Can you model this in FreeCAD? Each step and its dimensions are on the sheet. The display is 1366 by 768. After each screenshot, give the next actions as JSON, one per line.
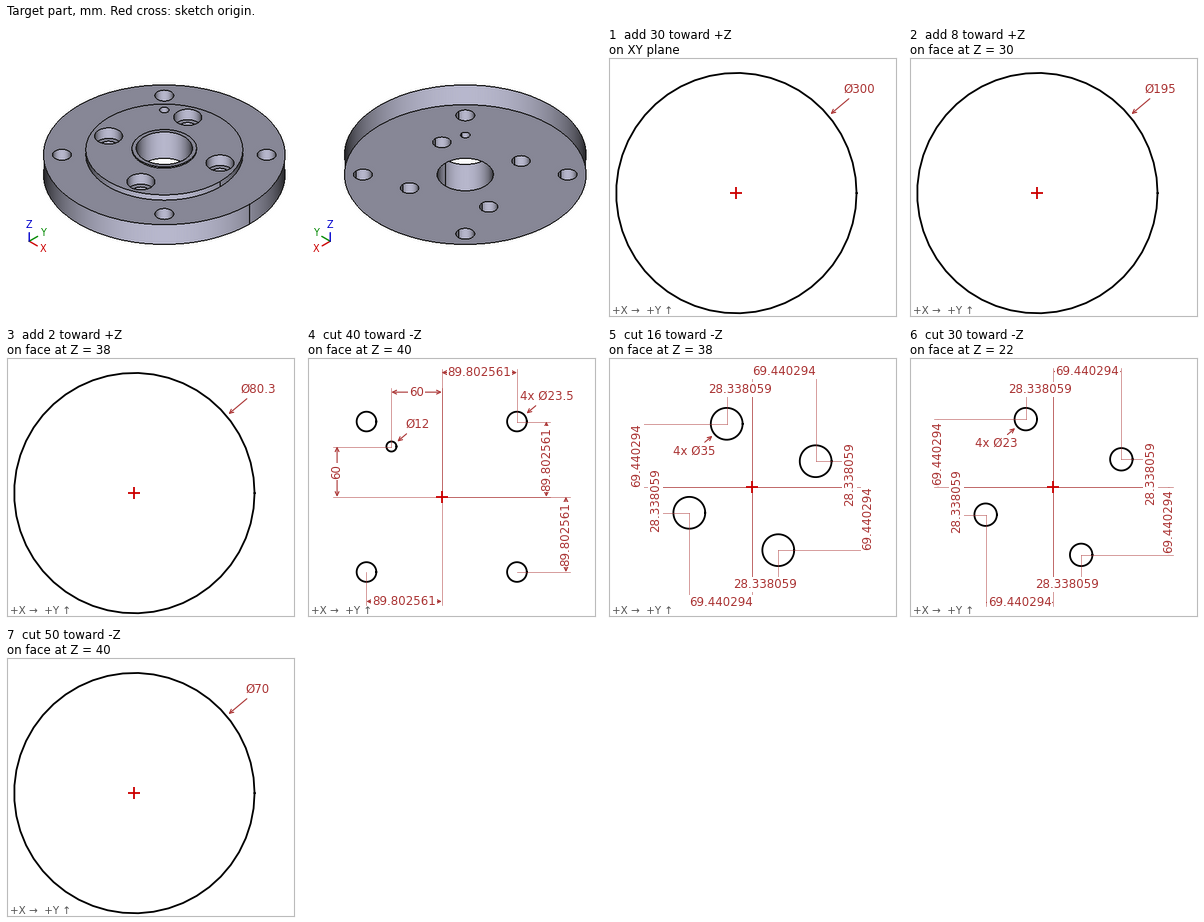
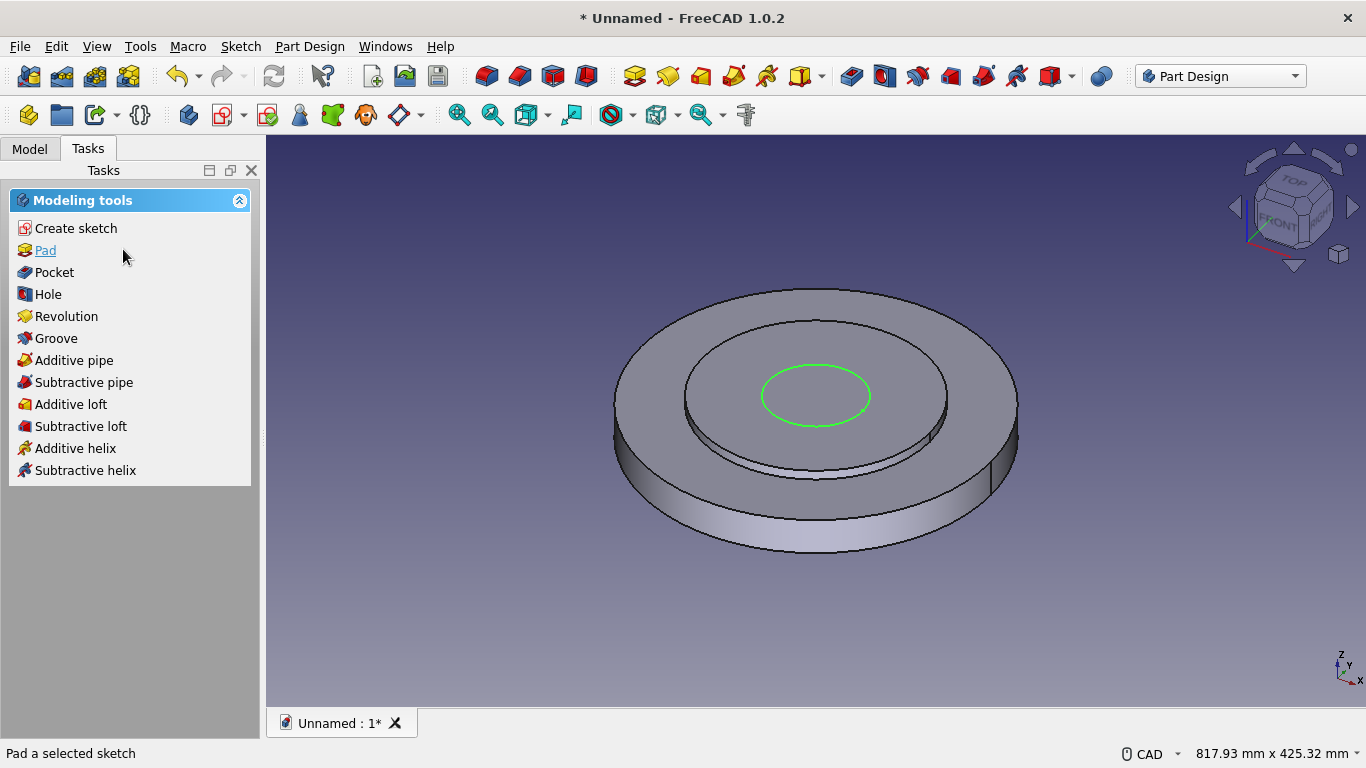
{"action": "left_click", "coordinate": [635, 76]}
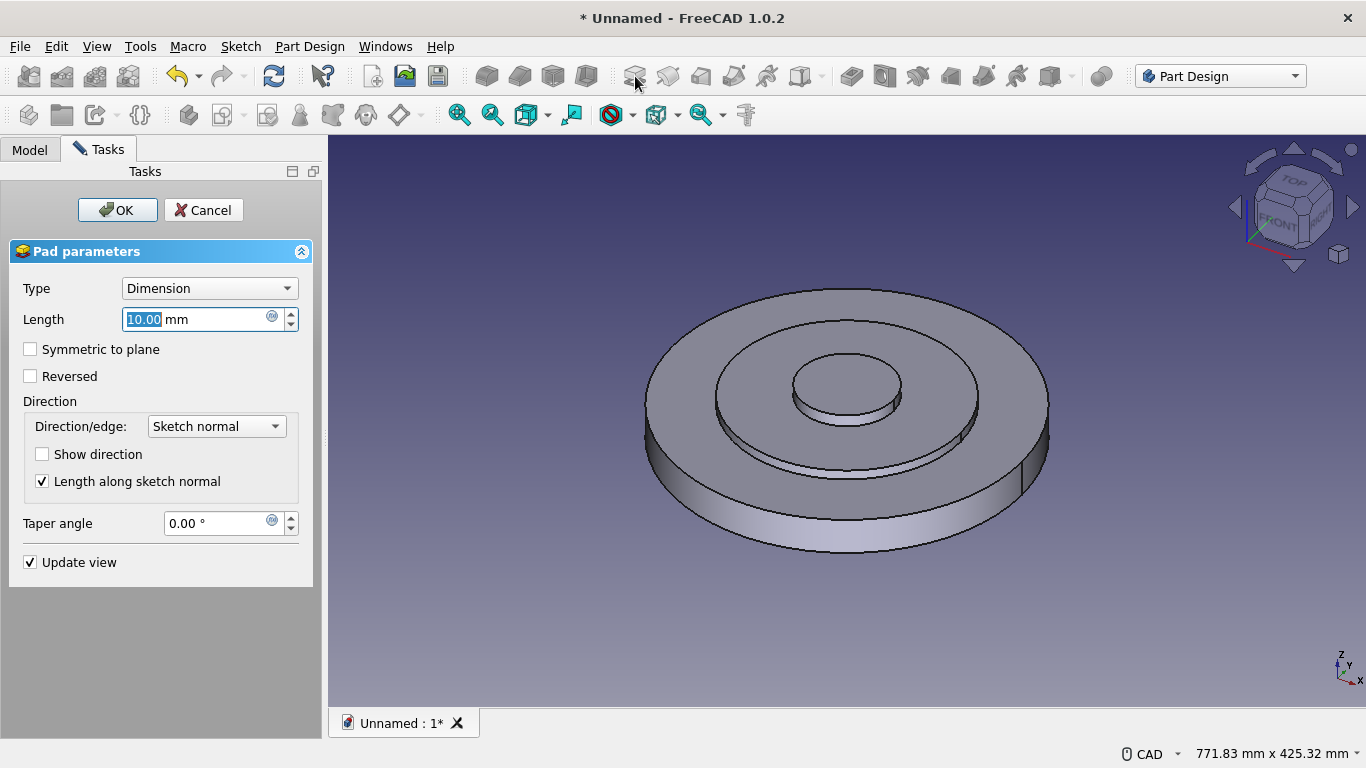
{"action": "type", "text": "2"}
{"action": "key", "text": "Tab"}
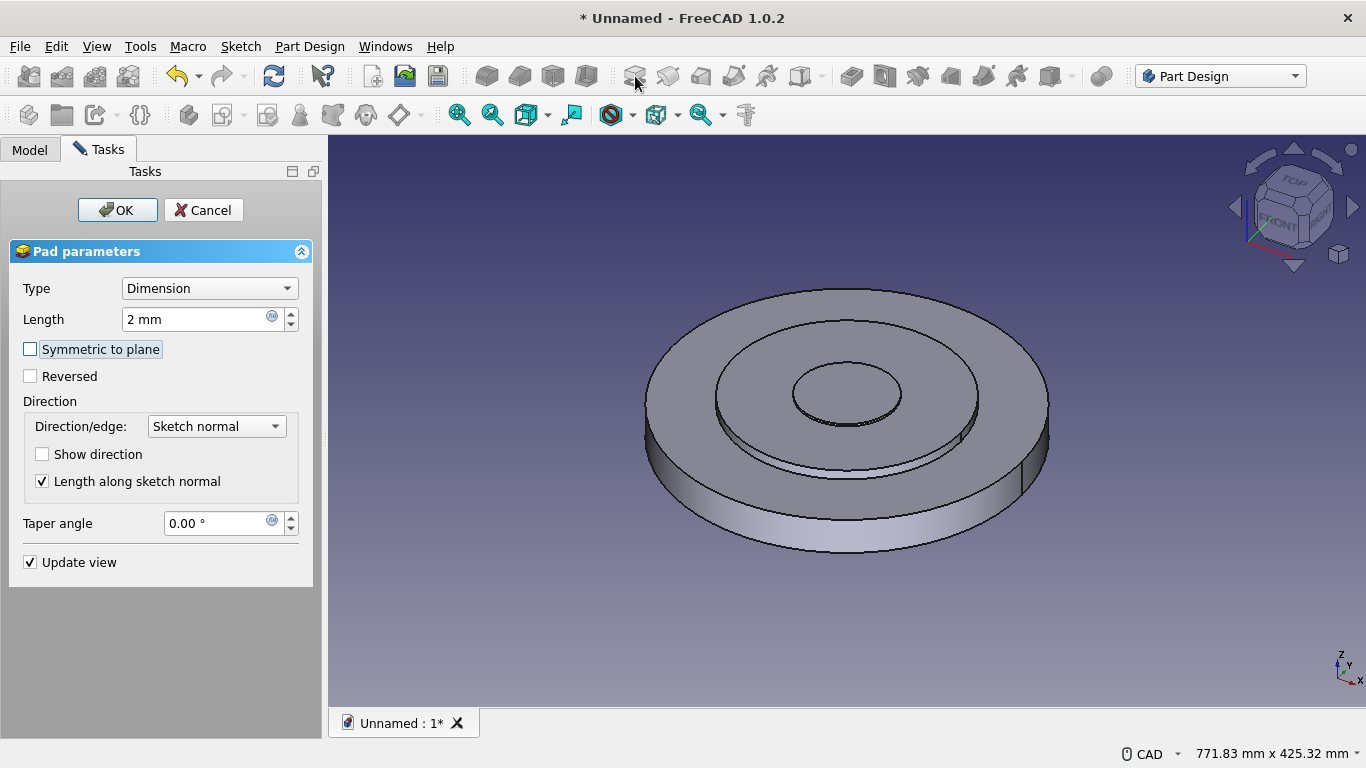
{"action": "left_click", "coordinate": [118, 210]}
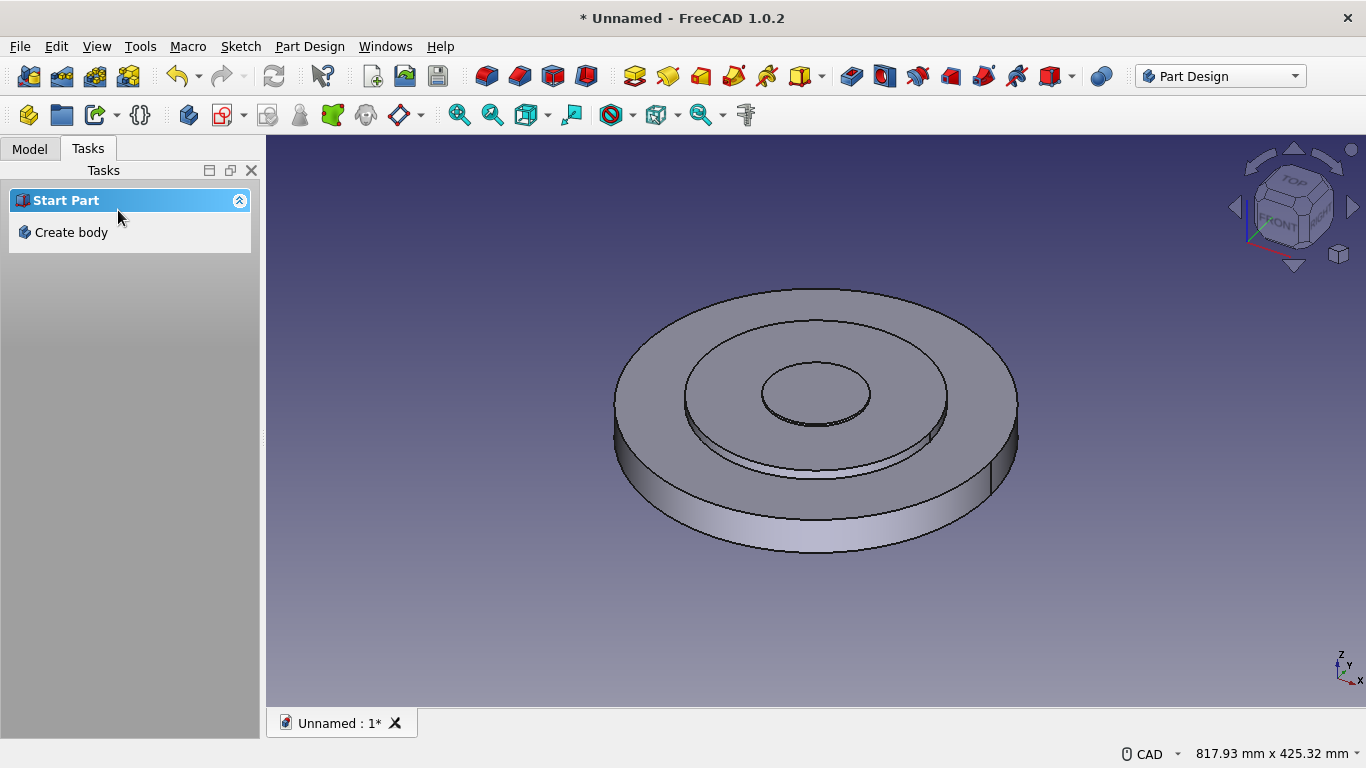
{"action": "left_click", "coordinate": [816, 392]}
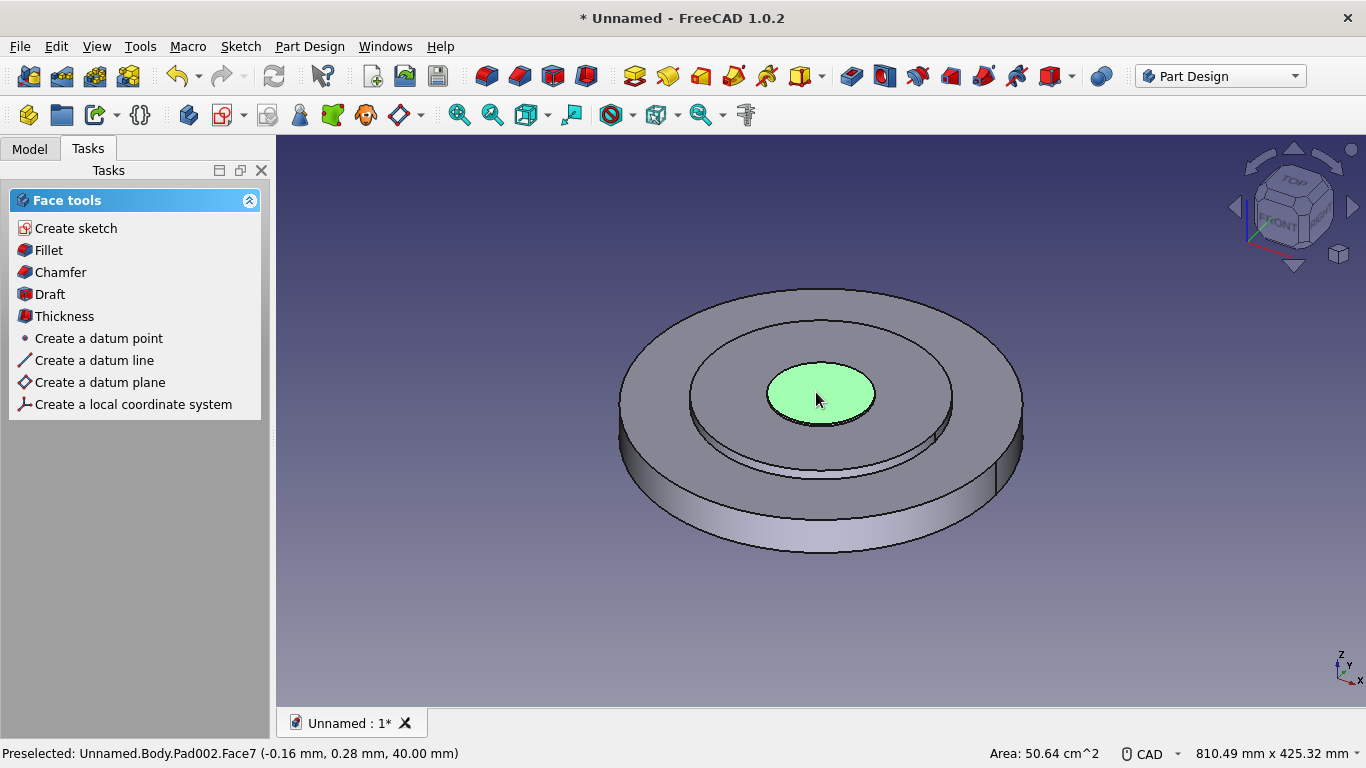
{"action": "left_click", "coordinate": [222, 116]}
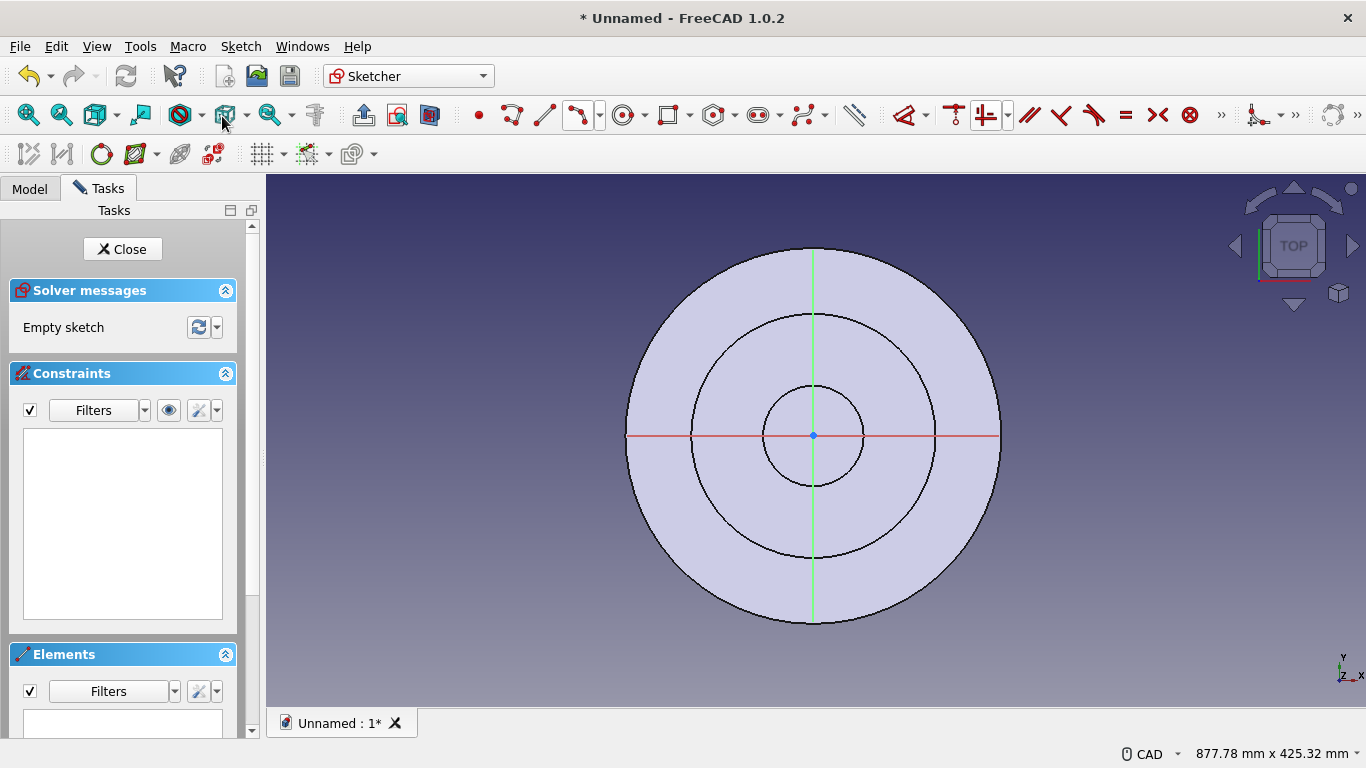
{"action": "left_click", "coordinate": [622, 116]}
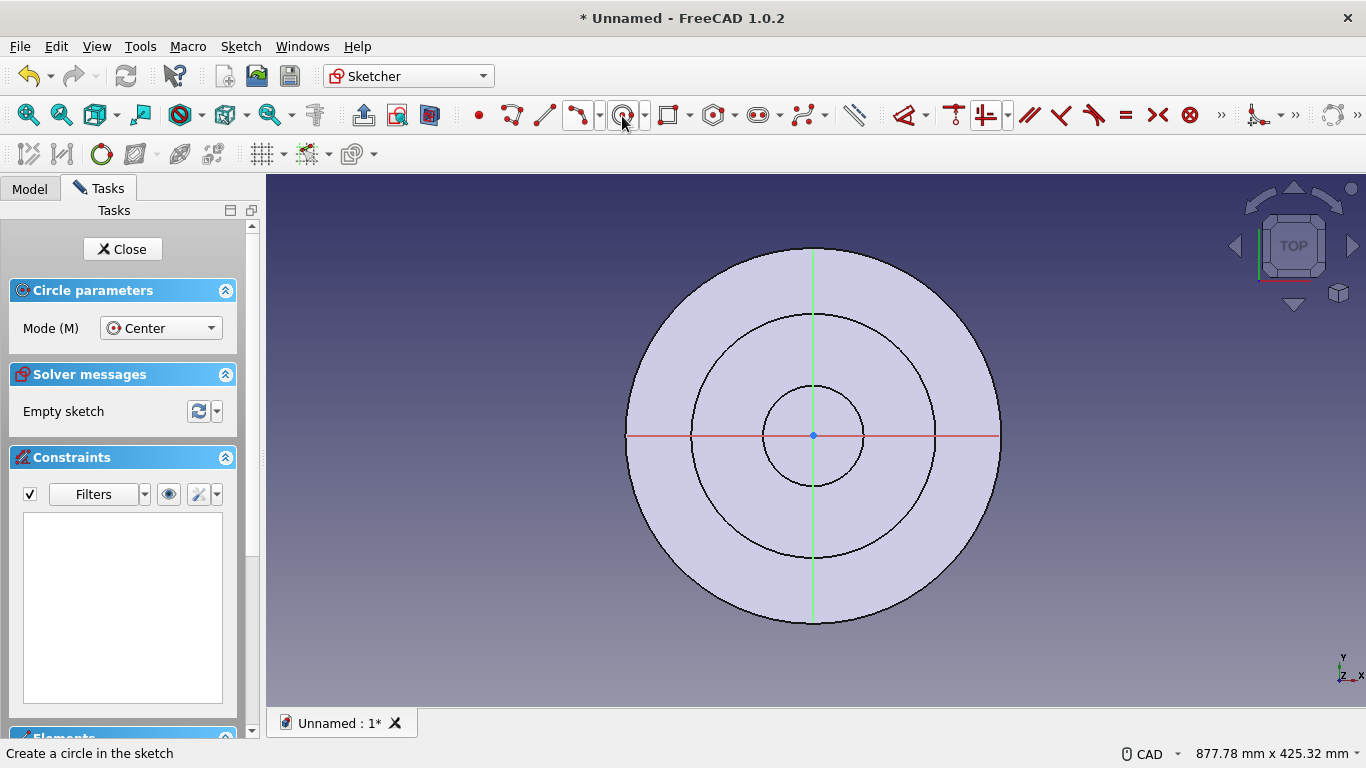
{"action": "scroll", "coordinate": [738, 361], "scroll_direction": "up", "scroll_amount": 6}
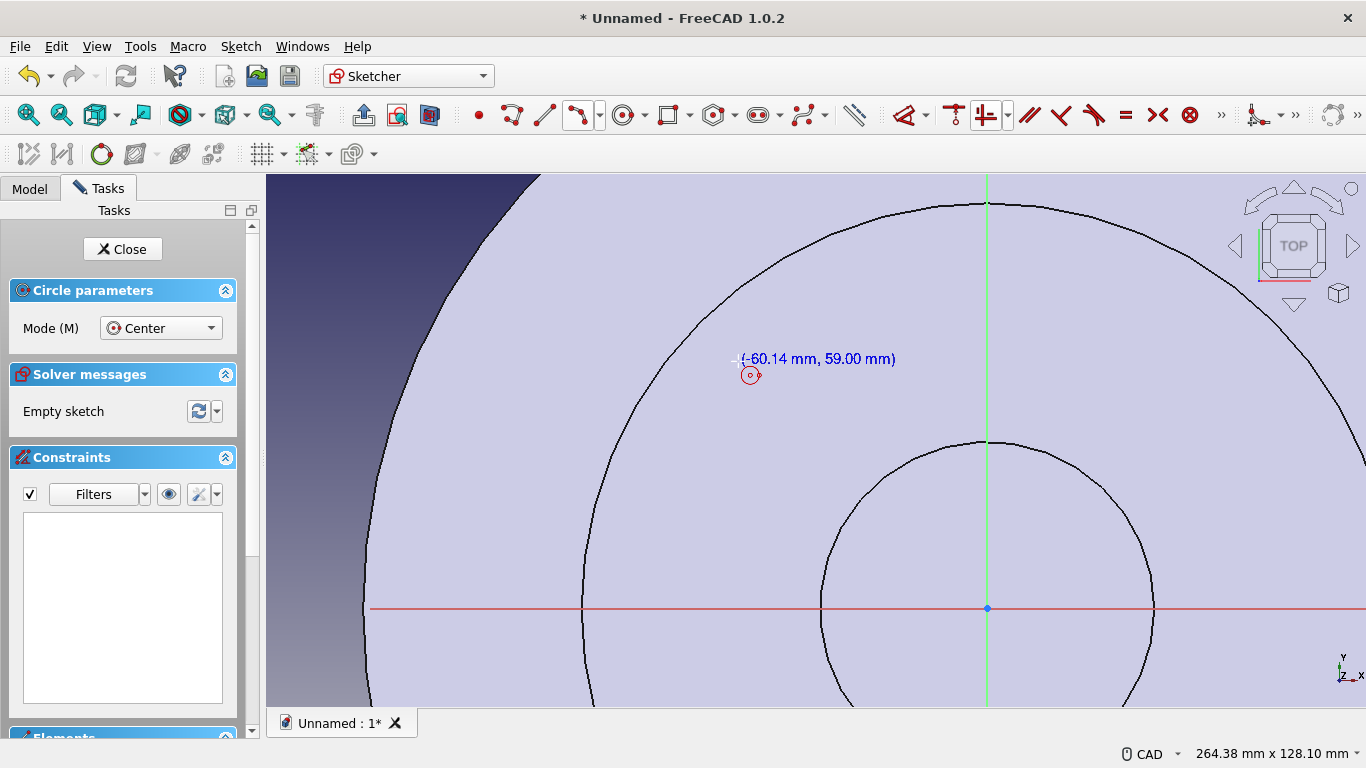
{"action": "left_click", "coordinate": [738, 359]}
{"action": "left_click", "coordinate": [755, 342]}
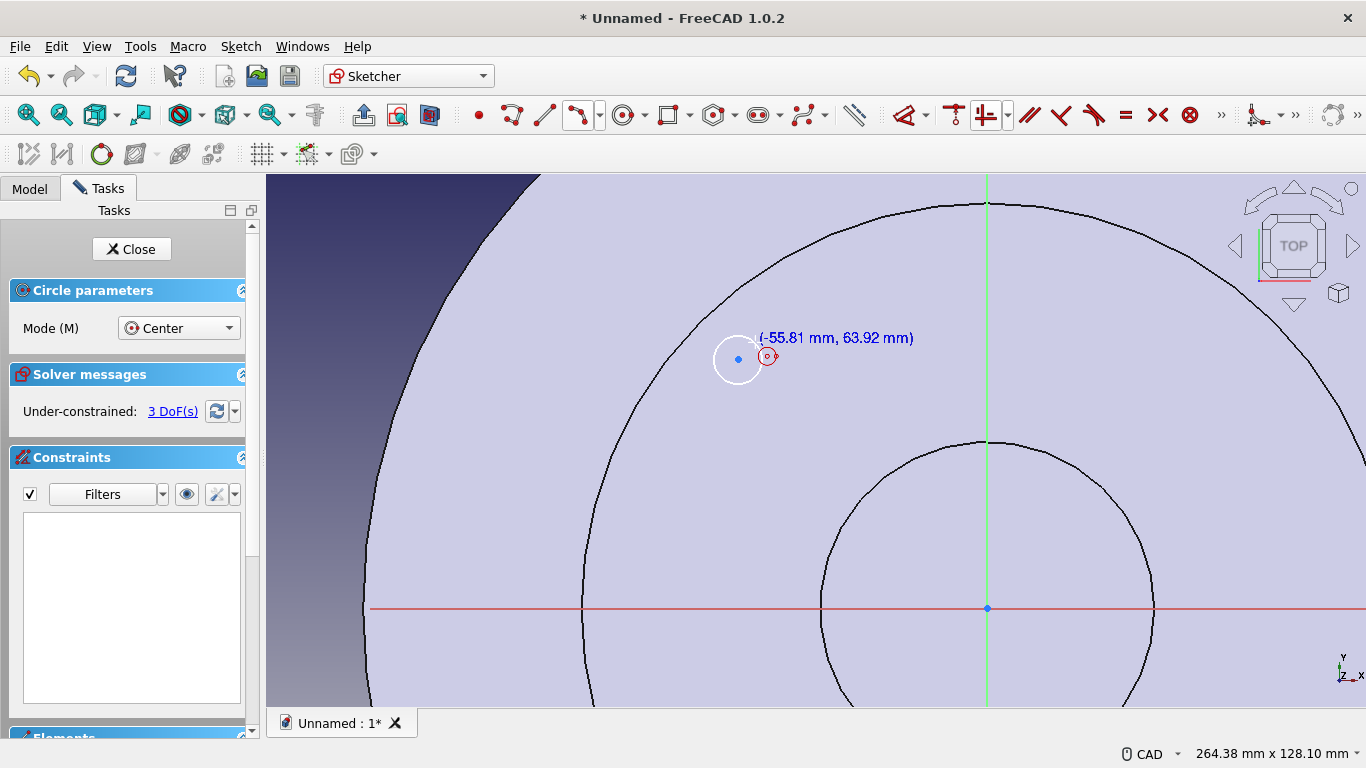
{"action": "scroll", "coordinate": [608, 342], "scroll_direction": "down", "scroll_amount": 5}